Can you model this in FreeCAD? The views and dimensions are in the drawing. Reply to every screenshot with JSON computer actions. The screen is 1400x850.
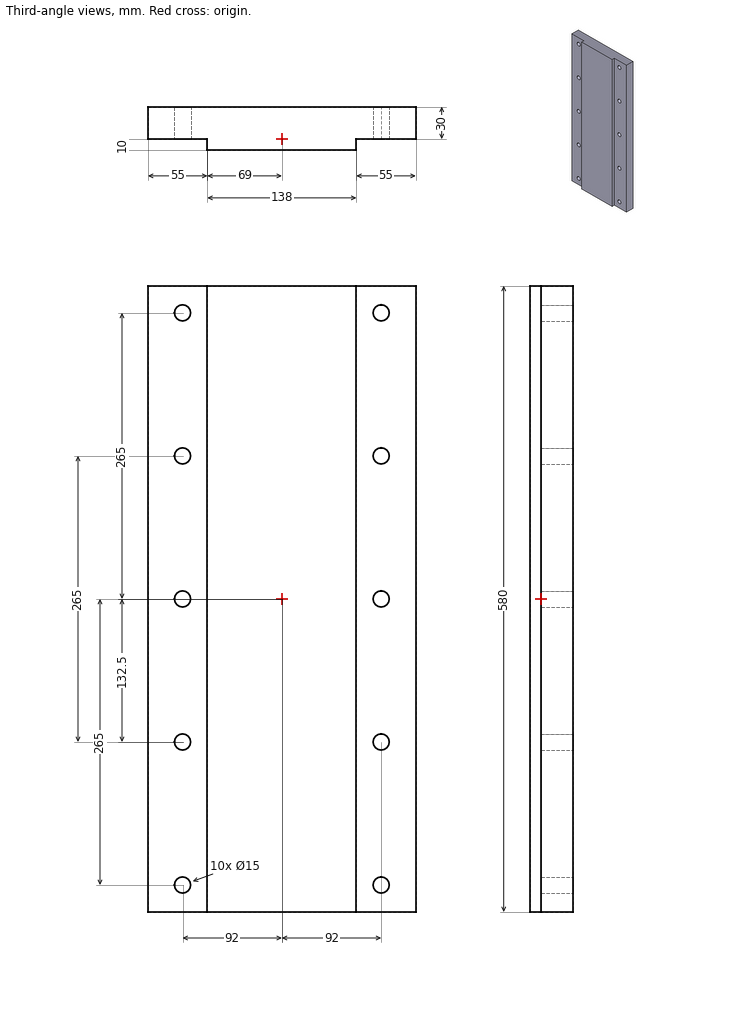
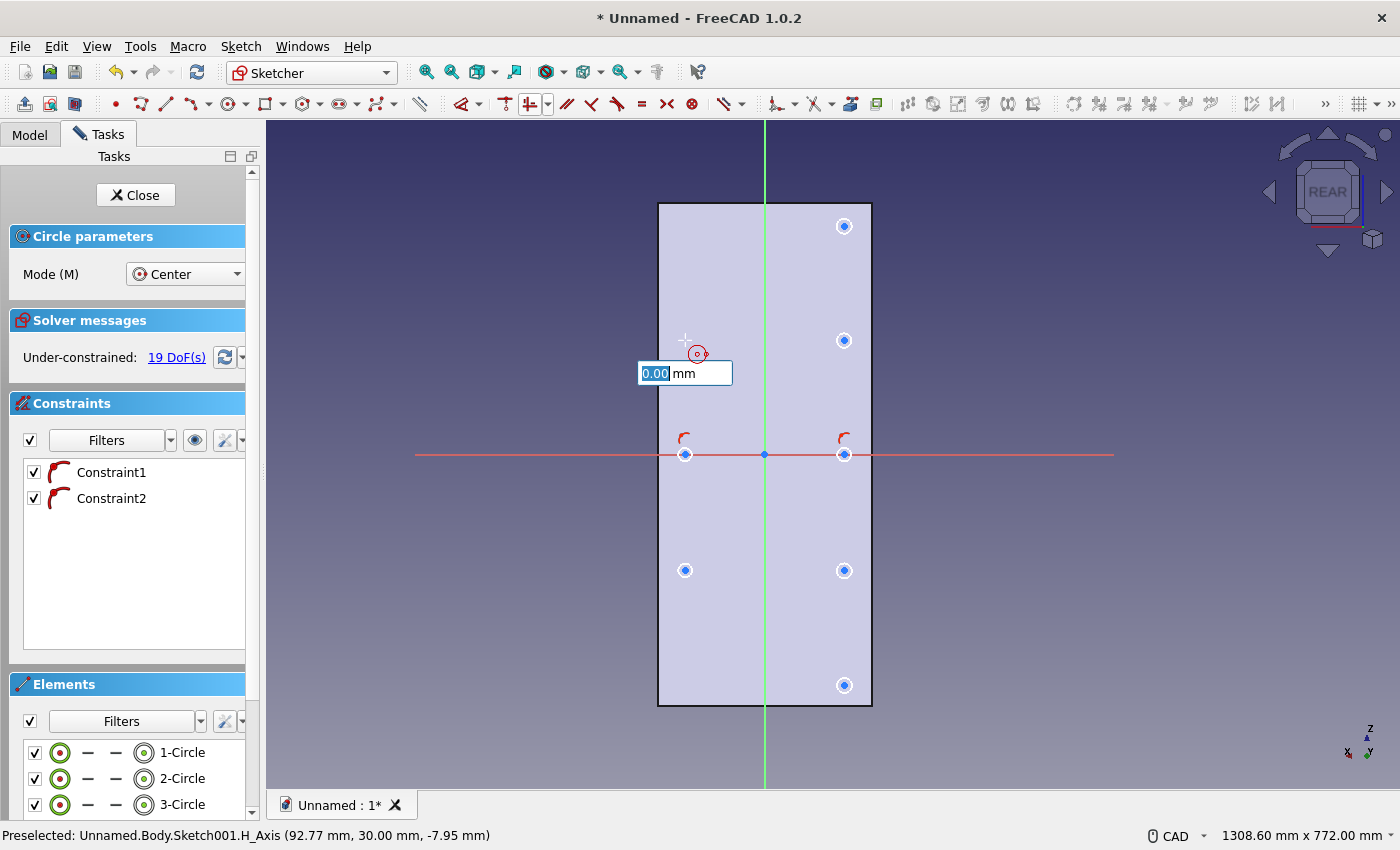
{"action": "scroll", "coordinate": [690, 335], "scroll_direction": "up", "scroll_amount": 5}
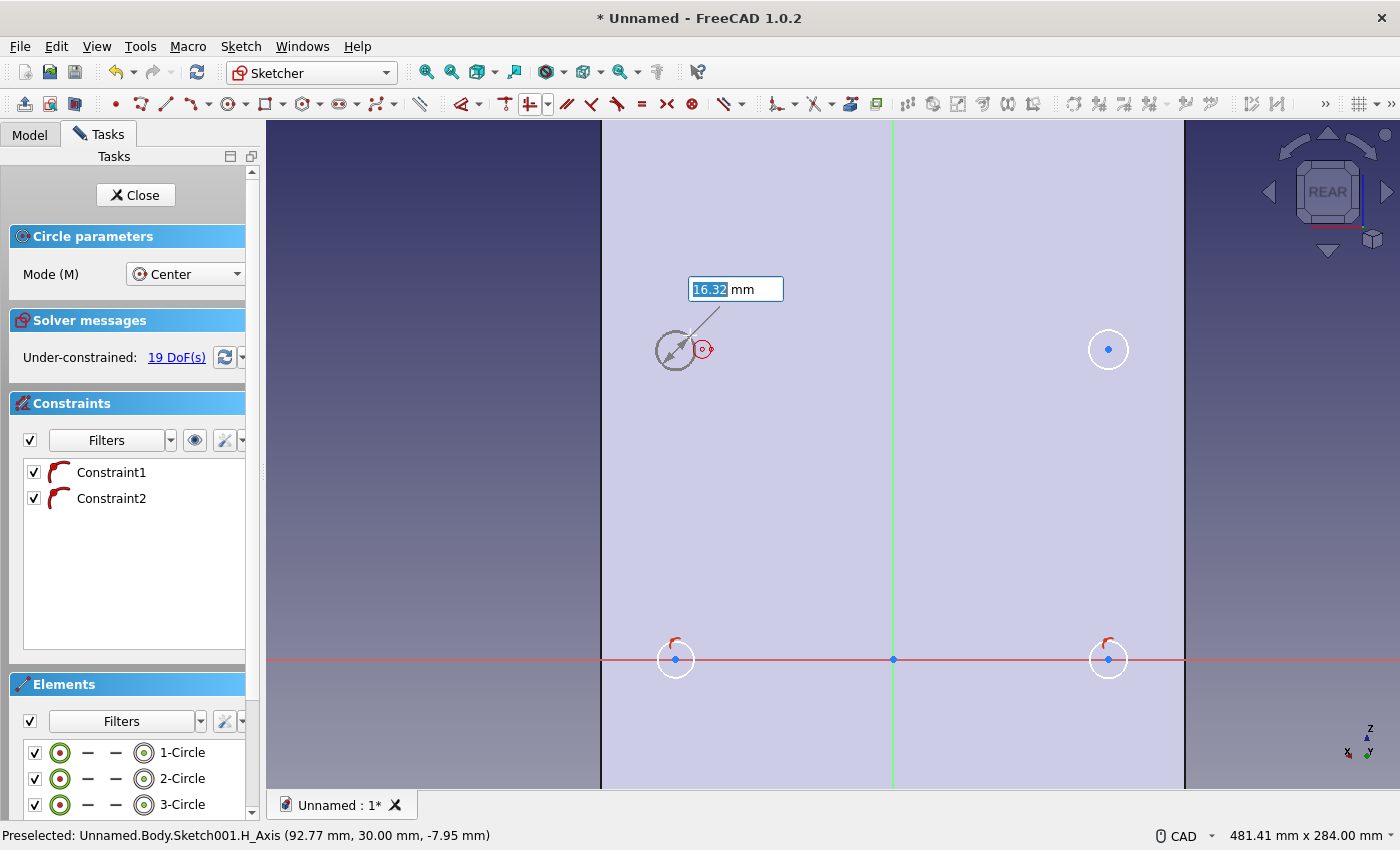
{"action": "left_click", "coordinate": [689, 335]}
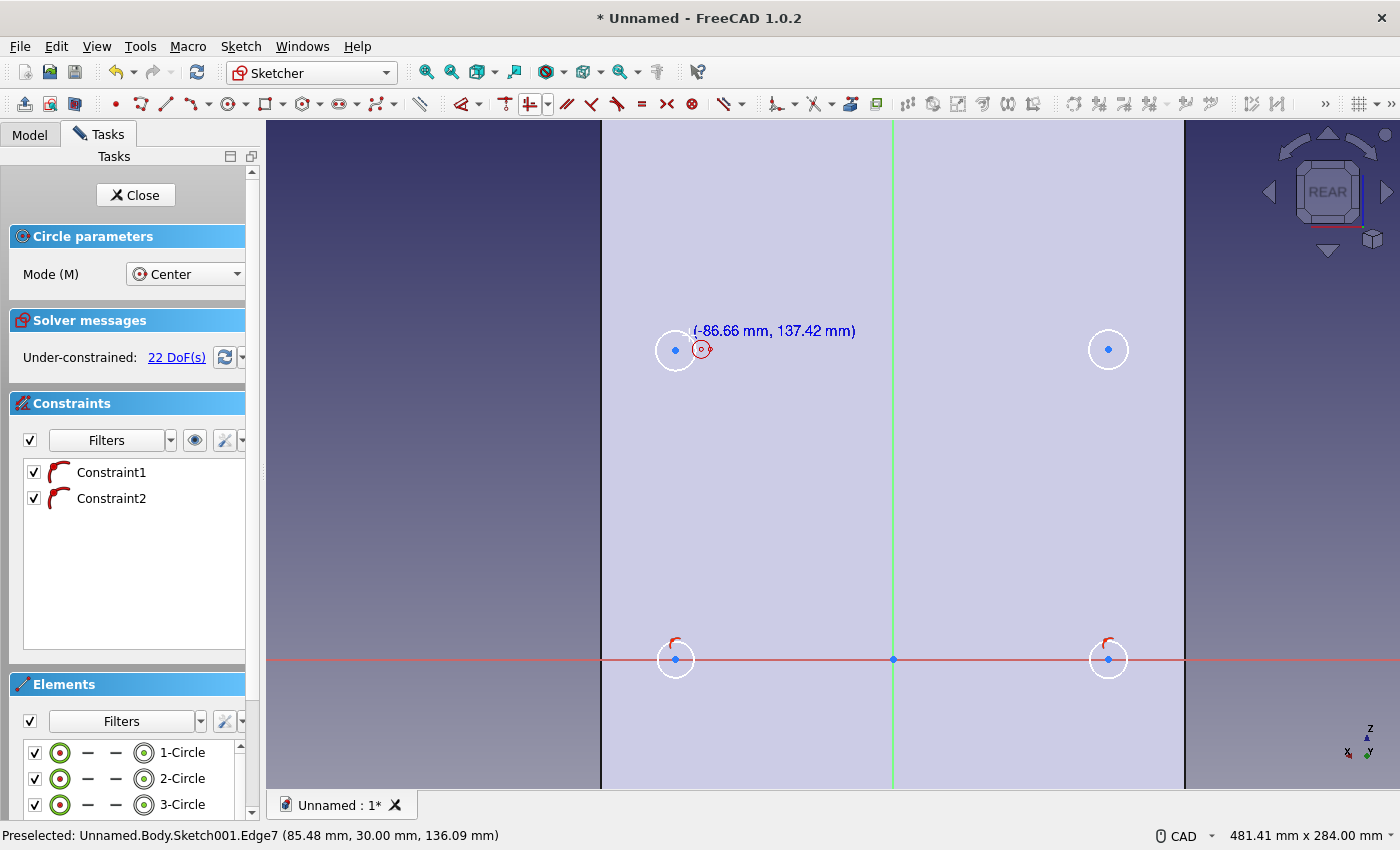
{"action": "scroll", "coordinate": [690, 335], "scroll_direction": "down", "scroll_amount": 5}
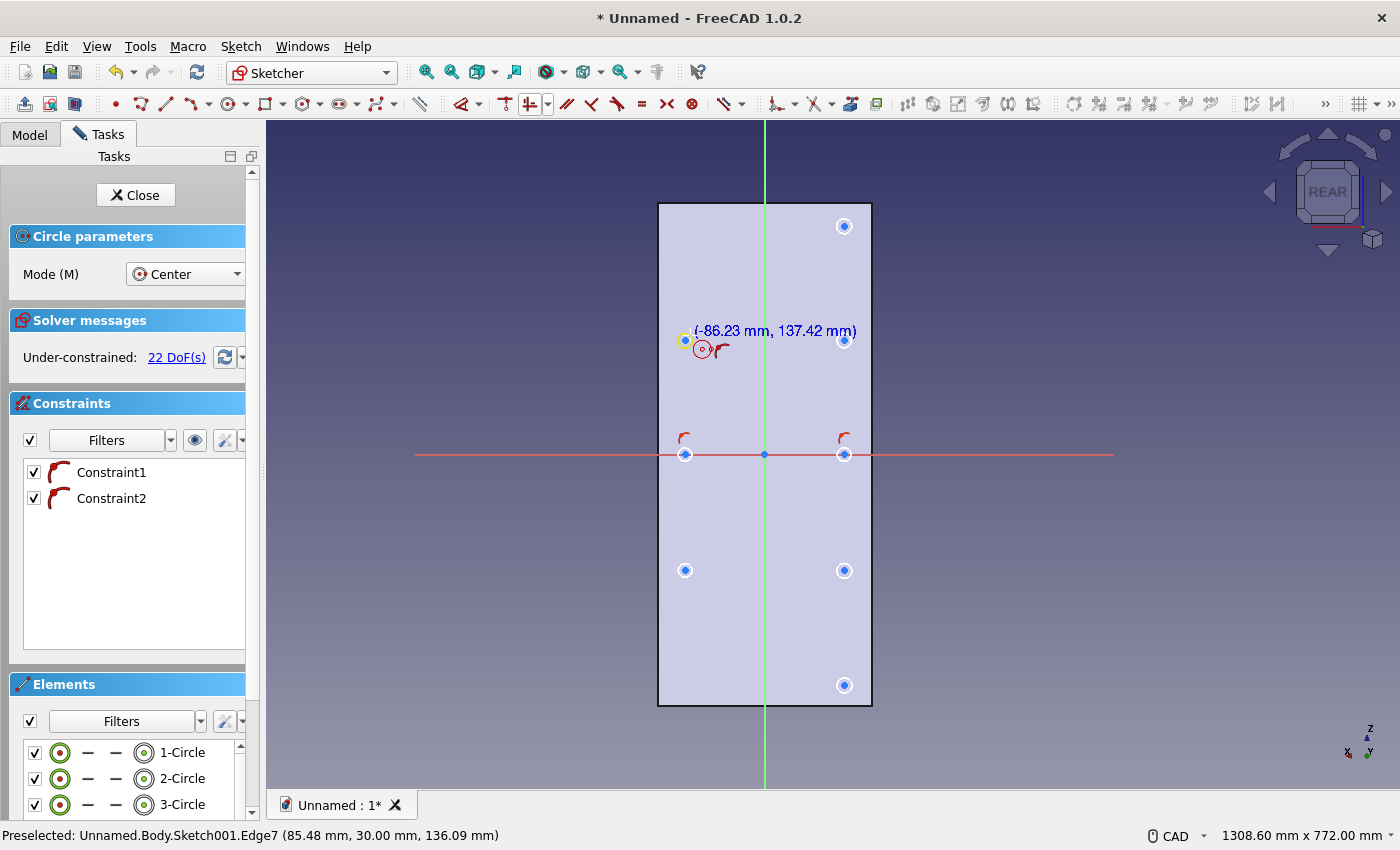
{"action": "scroll", "coordinate": [685, 225], "scroll_direction": "up", "scroll_amount": 7}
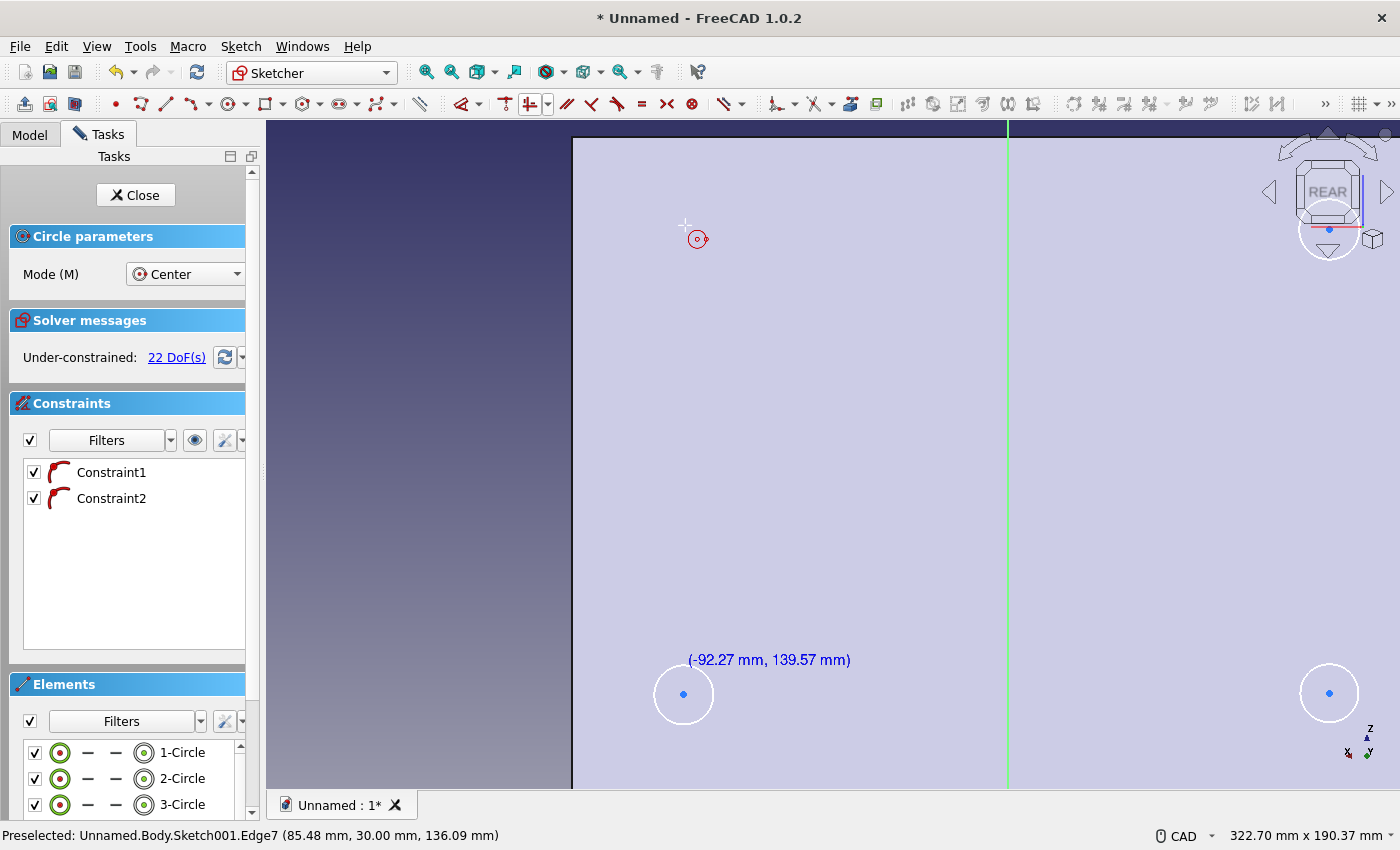
{"action": "scroll", "coordinate": [685, 225], "scroll_direction": "down", "scroll_amount": 7}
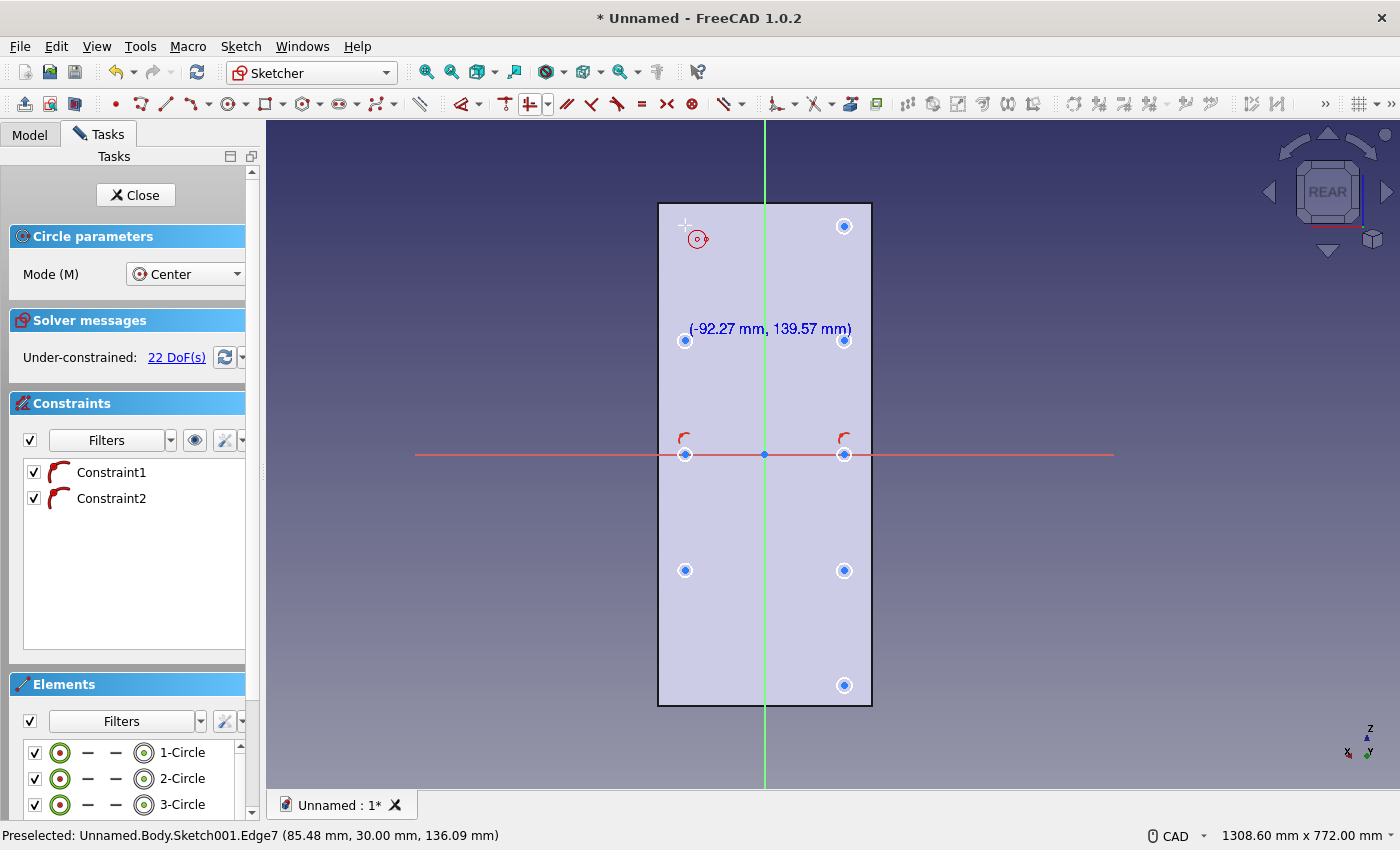
{"action": "left_click", "coordinate": [685, 225]}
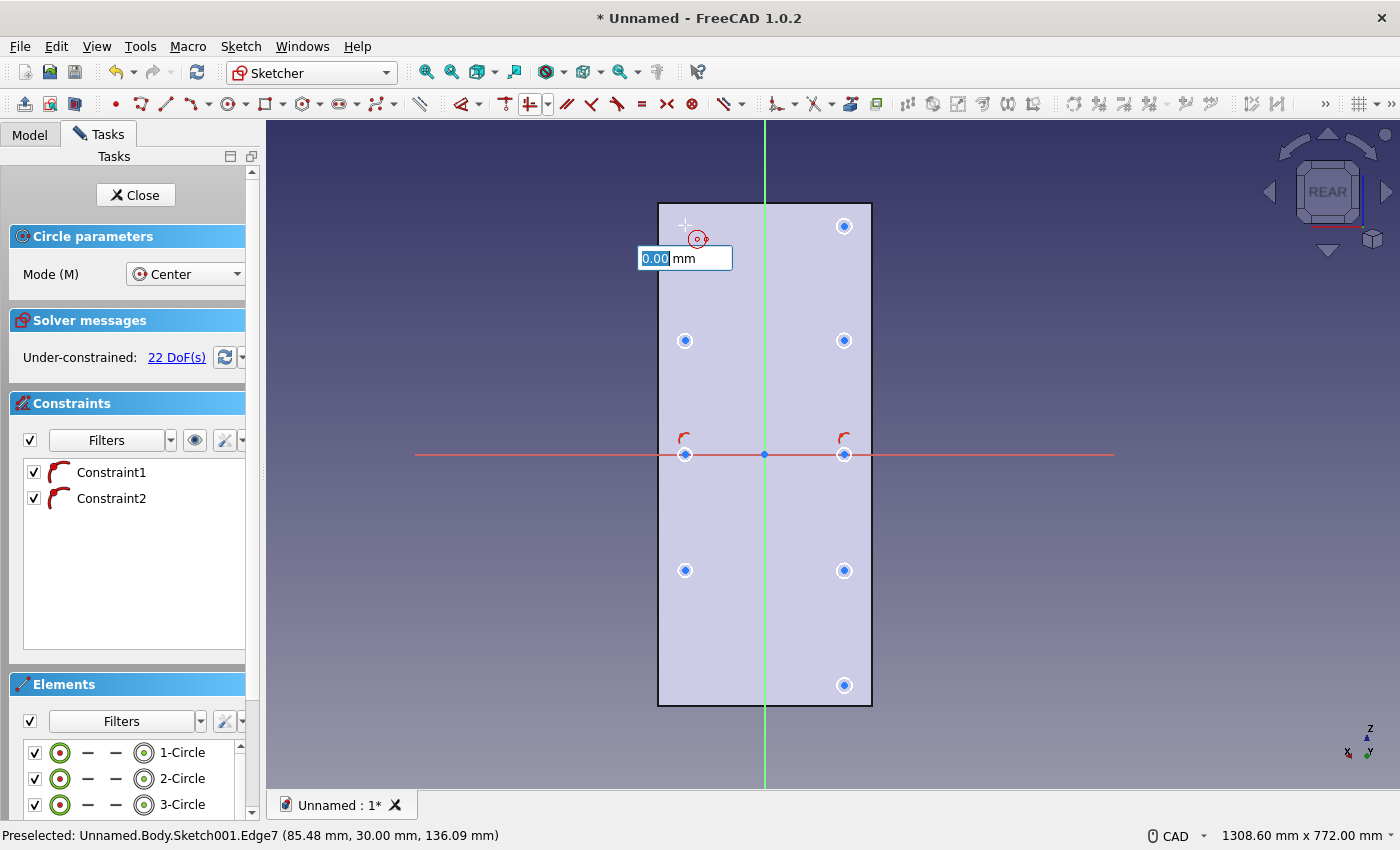
{"action": "scroll", "coordinate": [690, 220], "scroll_direction": "up", "scroll_amount": 5}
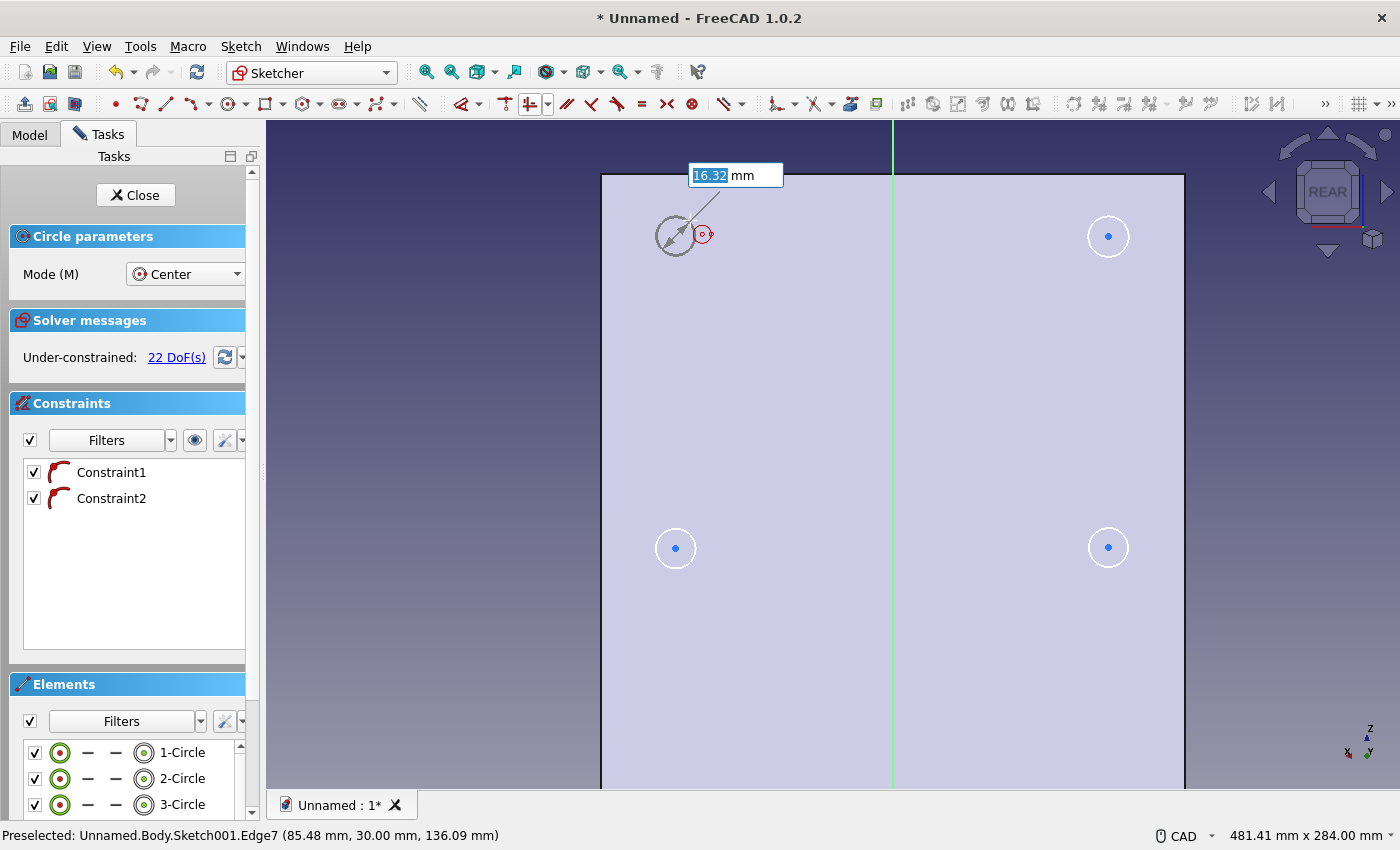
{"action": "left_click", "coordinate": [689, 221]}